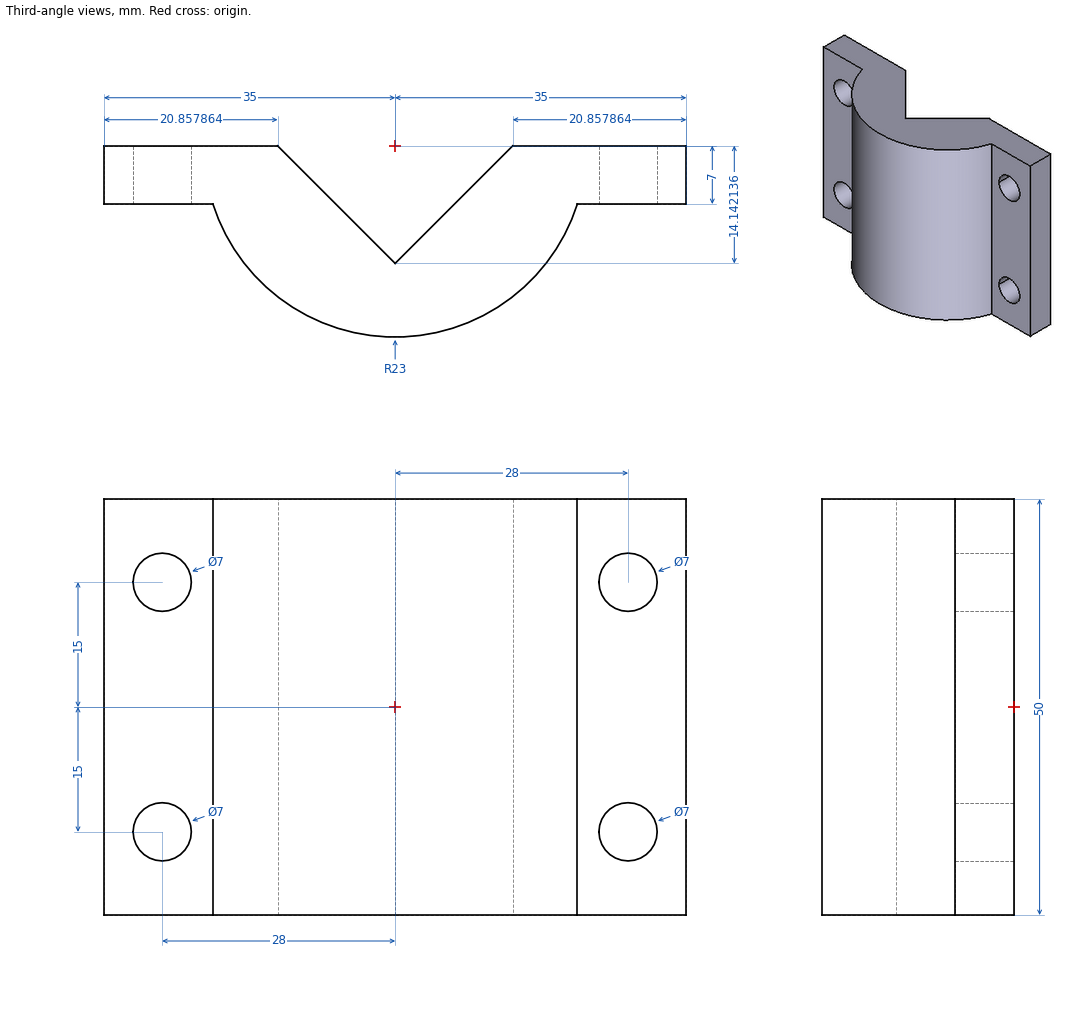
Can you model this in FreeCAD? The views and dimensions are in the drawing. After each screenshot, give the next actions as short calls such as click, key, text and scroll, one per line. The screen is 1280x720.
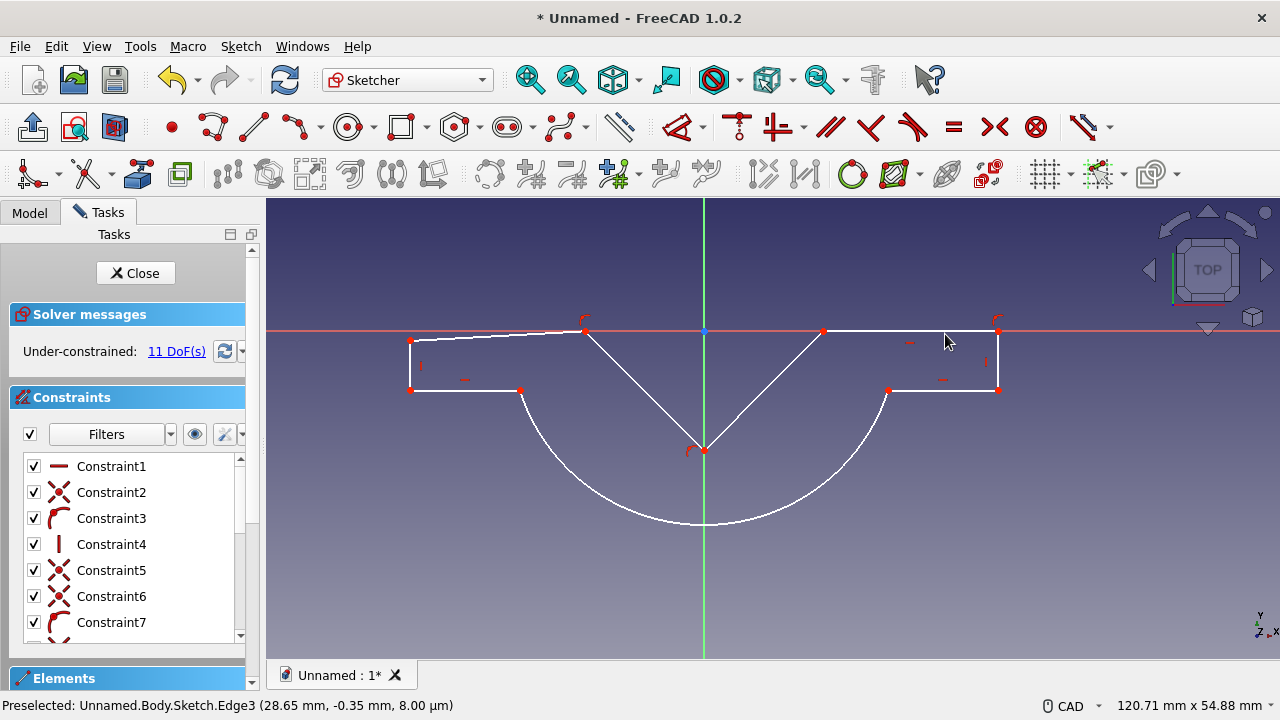
click(533, 334)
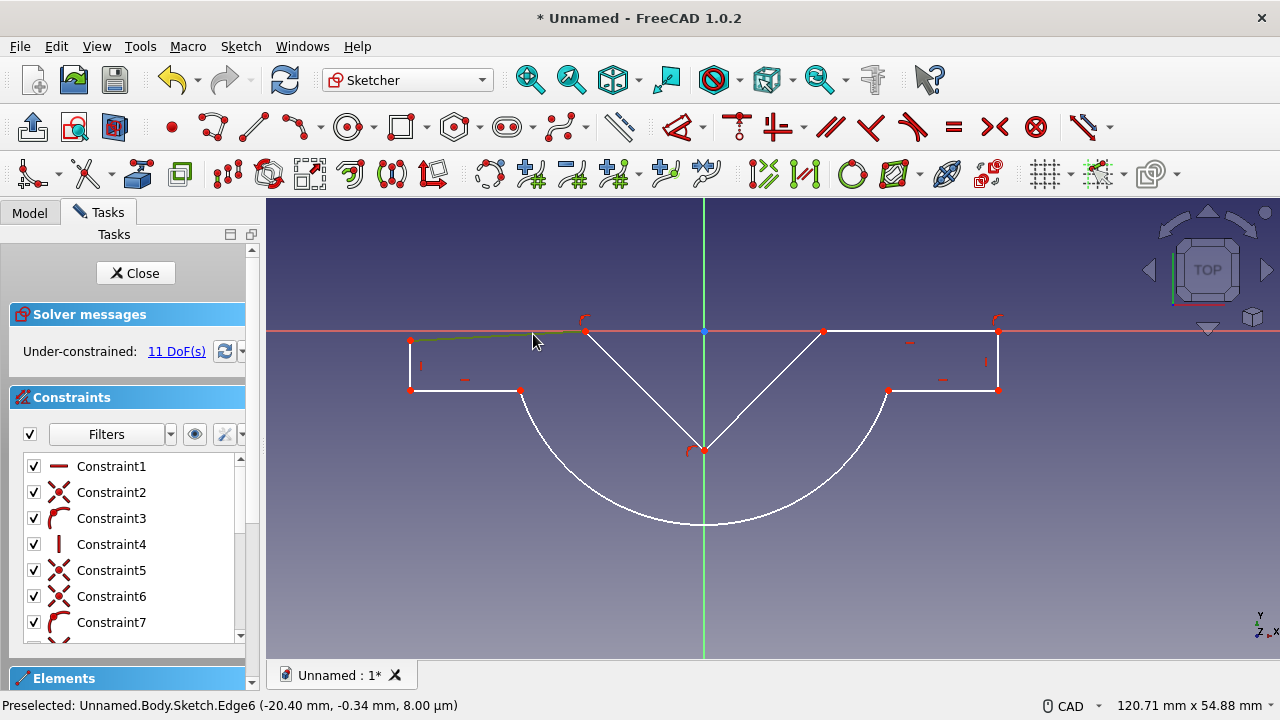
key(h)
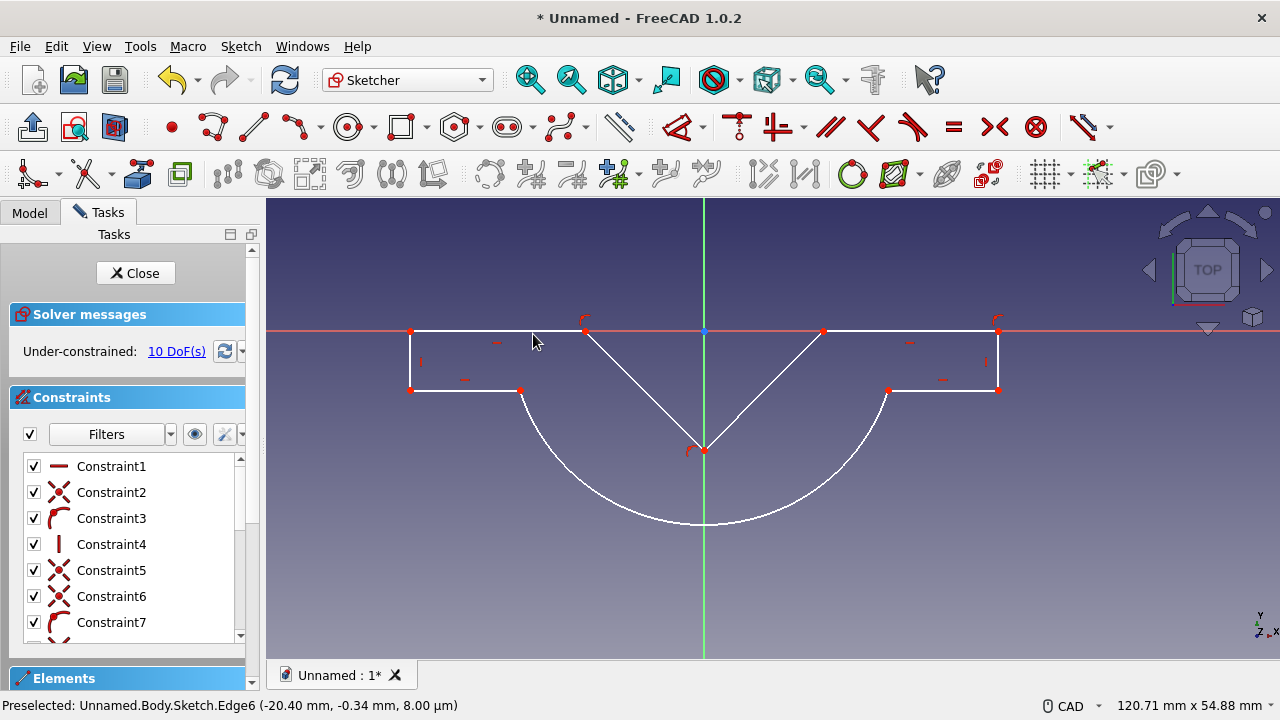
drag(694, 321, 714, 342)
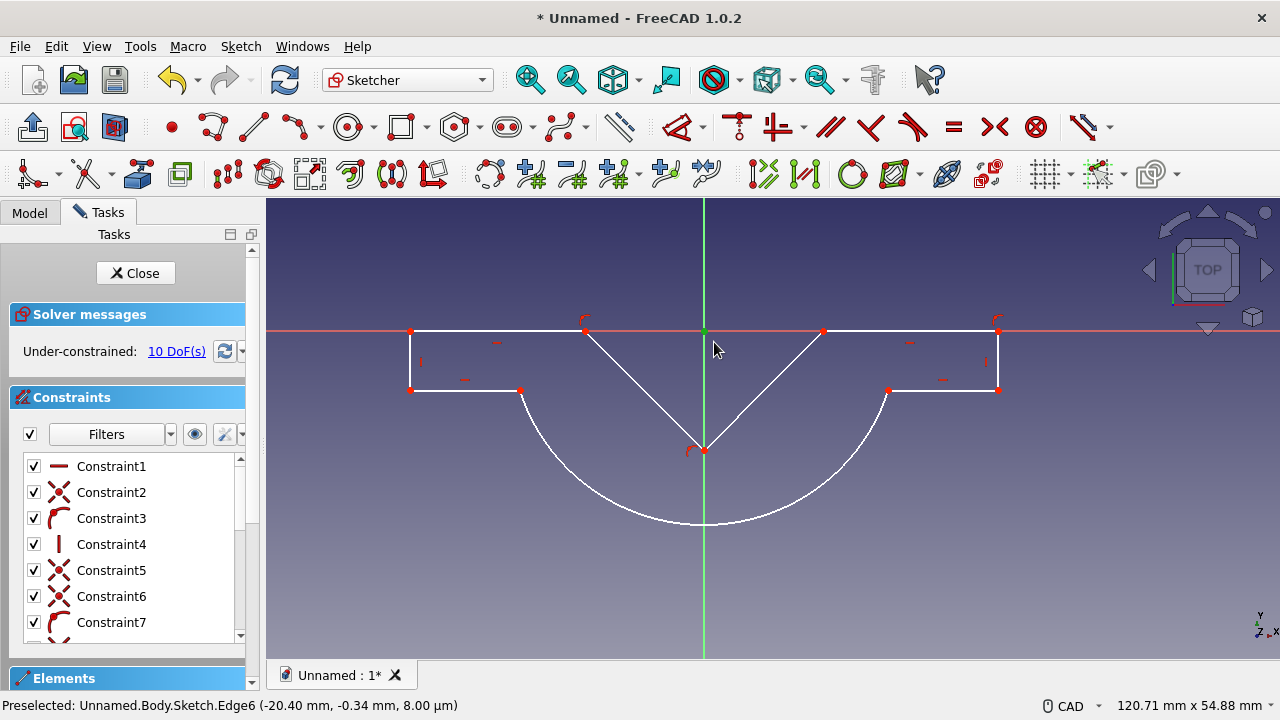
key(c)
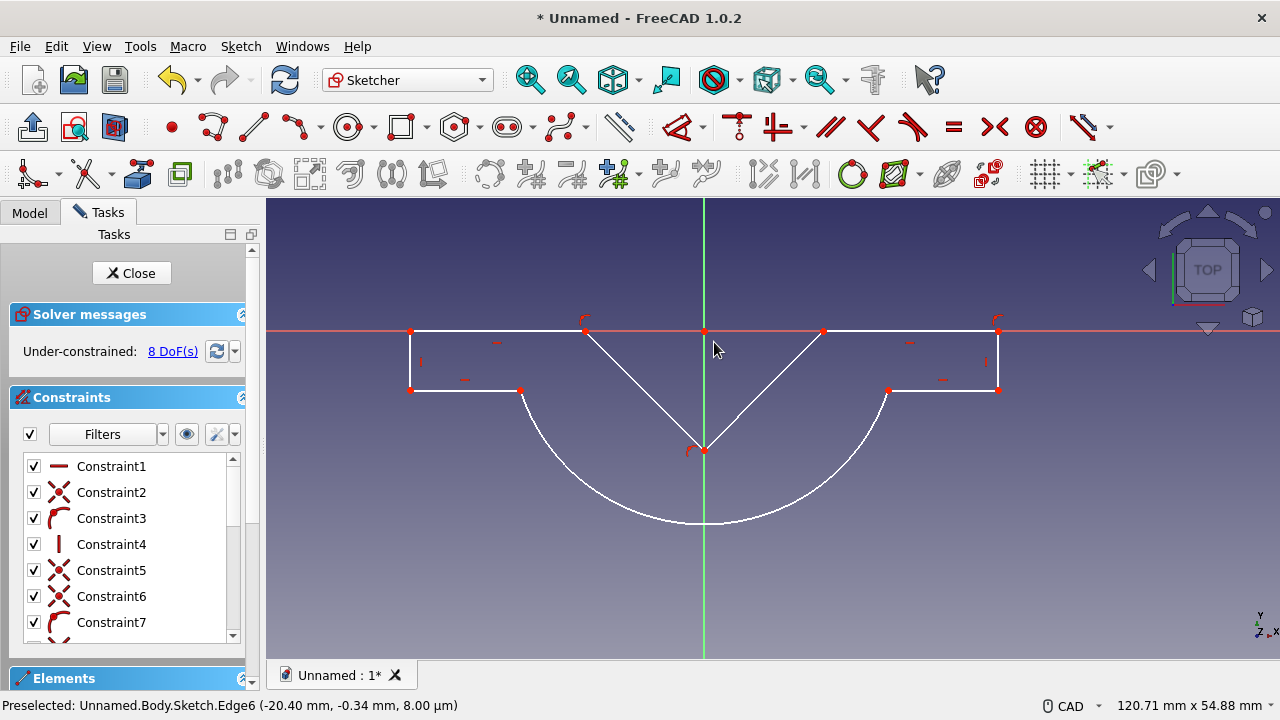
key(d)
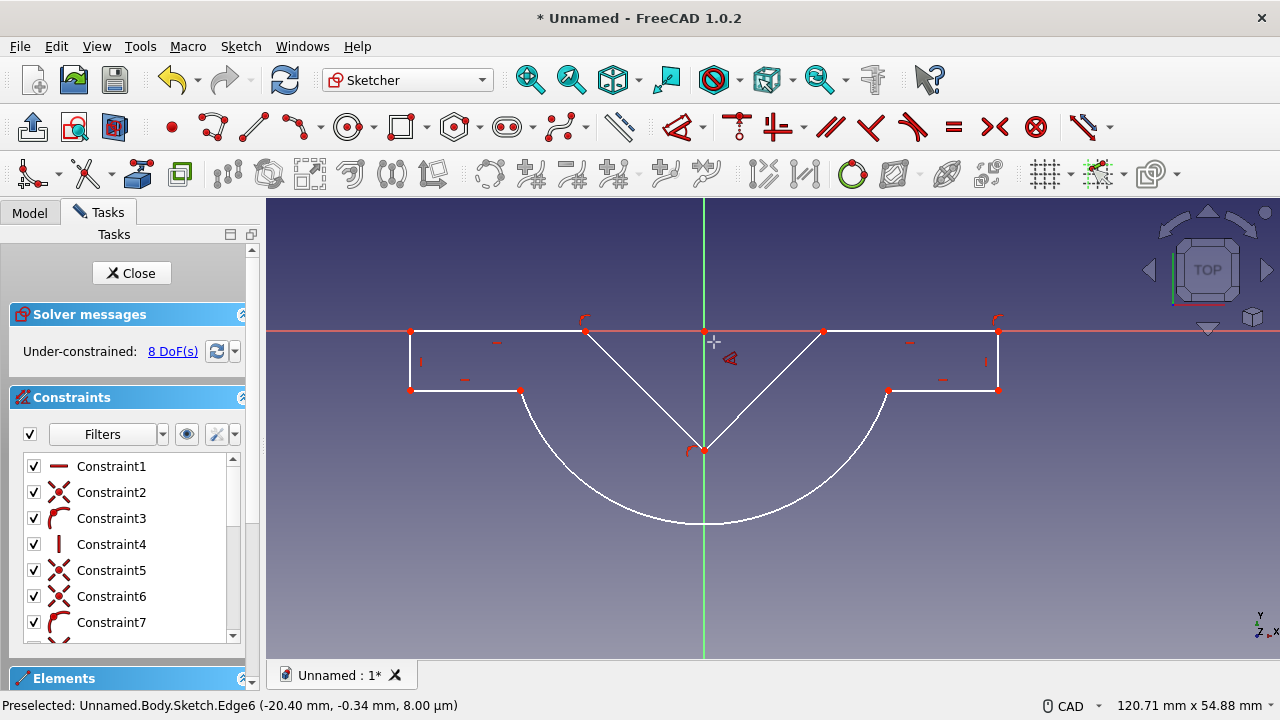
click(611, 501)
click(596, 529)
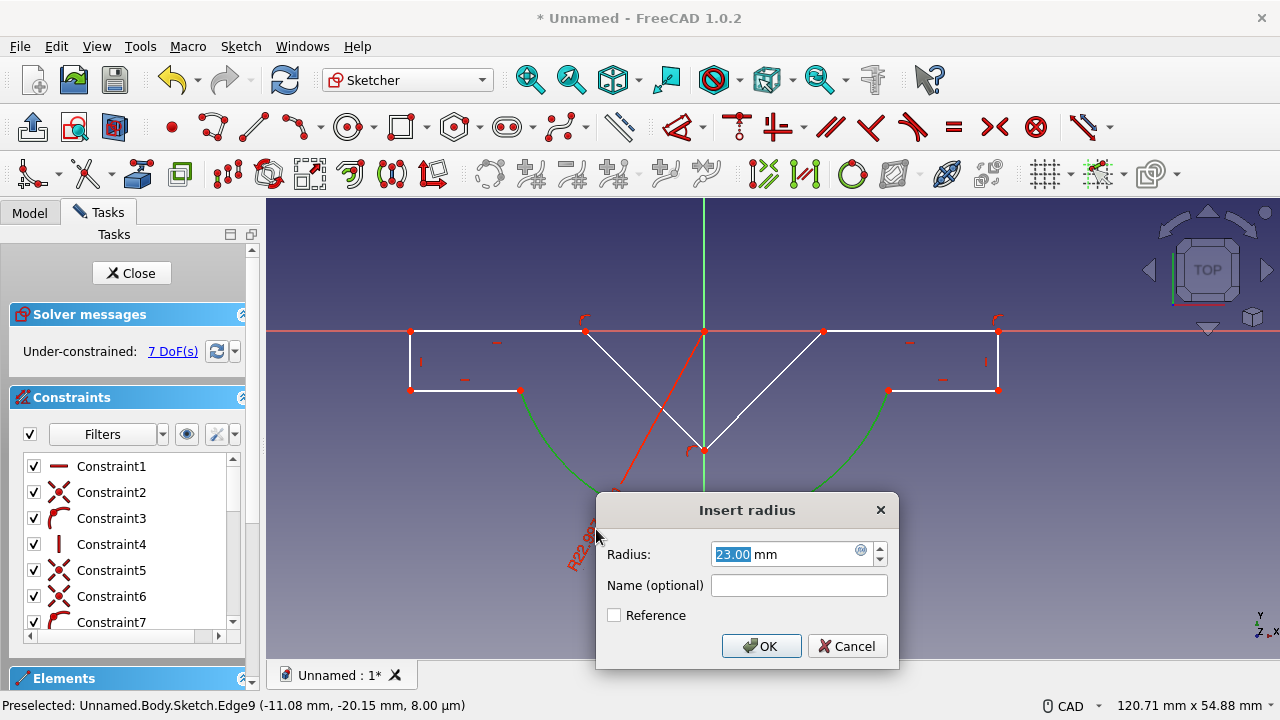
text(23)
key(Return)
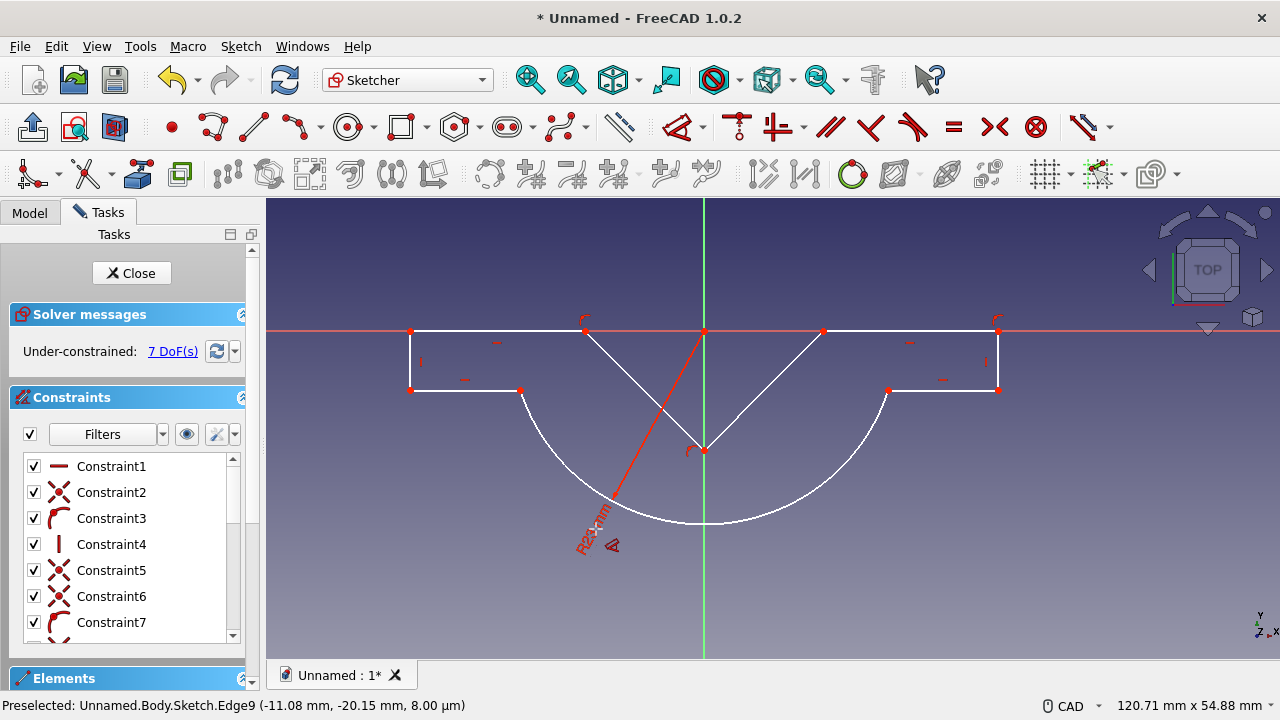
click(998, 373)
click(1032, 361)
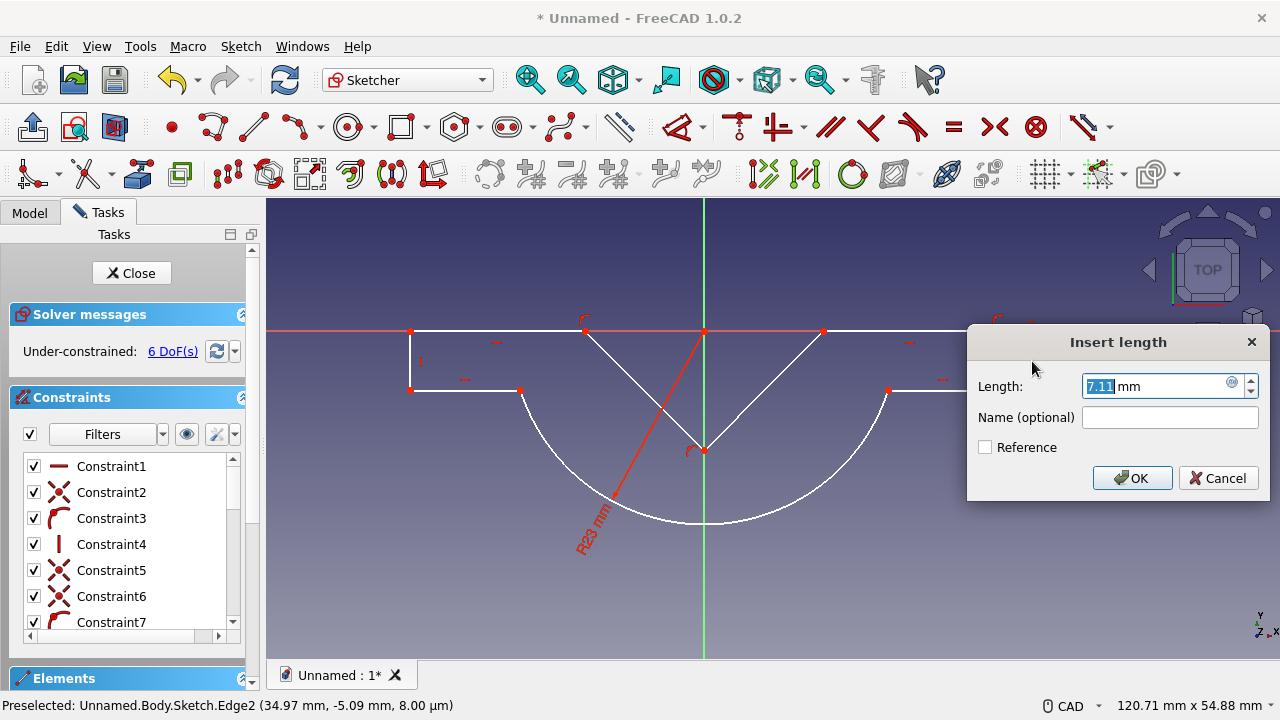
text(7)
key(Return)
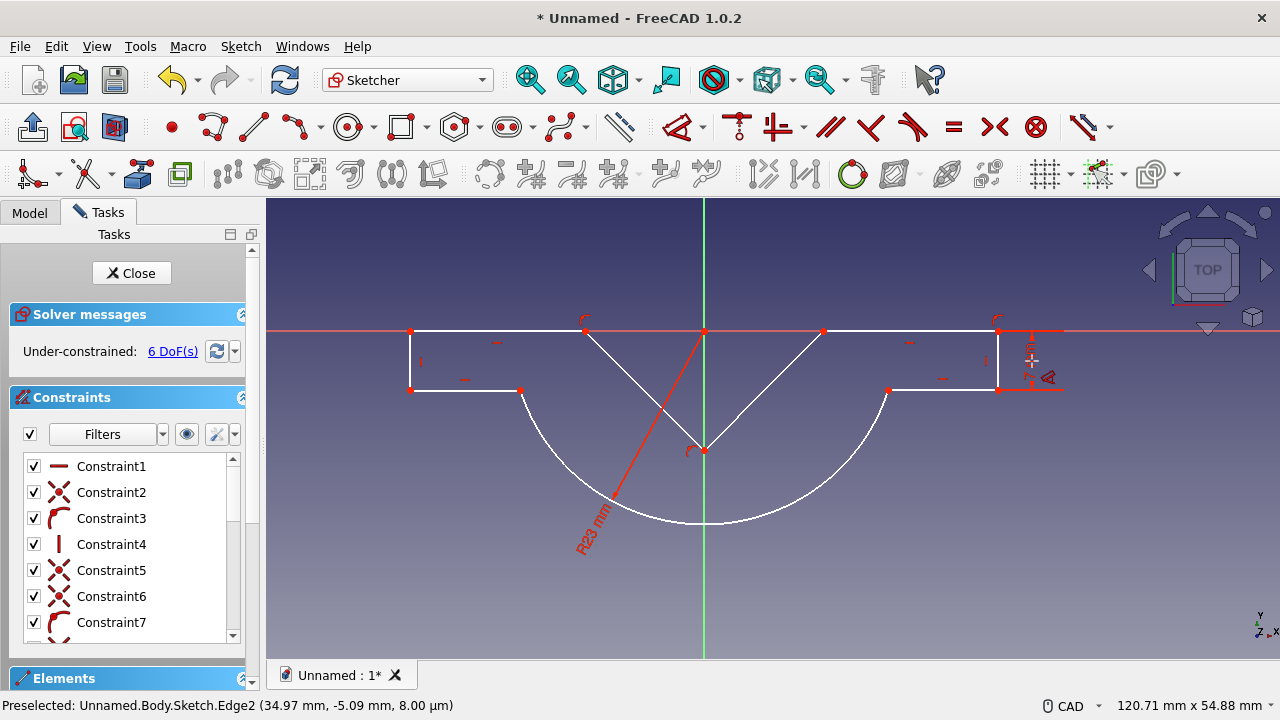
click(410, 349)
click(376, 361)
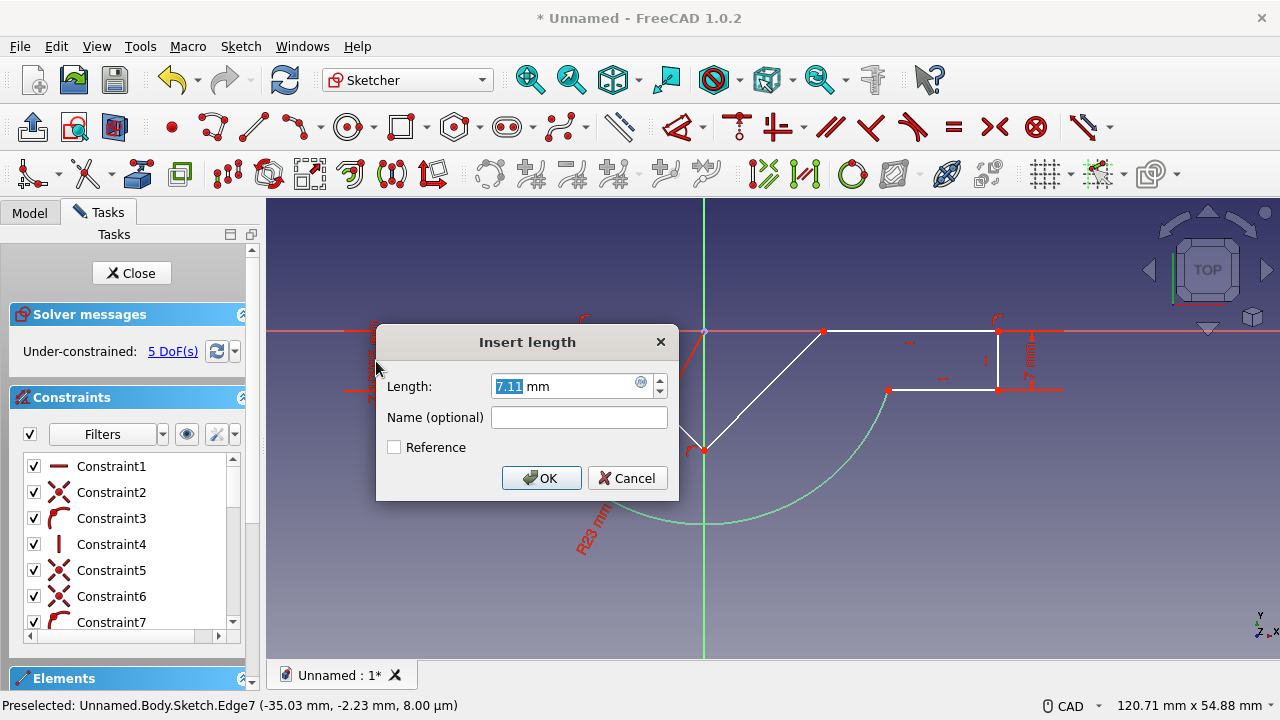
text(7)
key(Return)